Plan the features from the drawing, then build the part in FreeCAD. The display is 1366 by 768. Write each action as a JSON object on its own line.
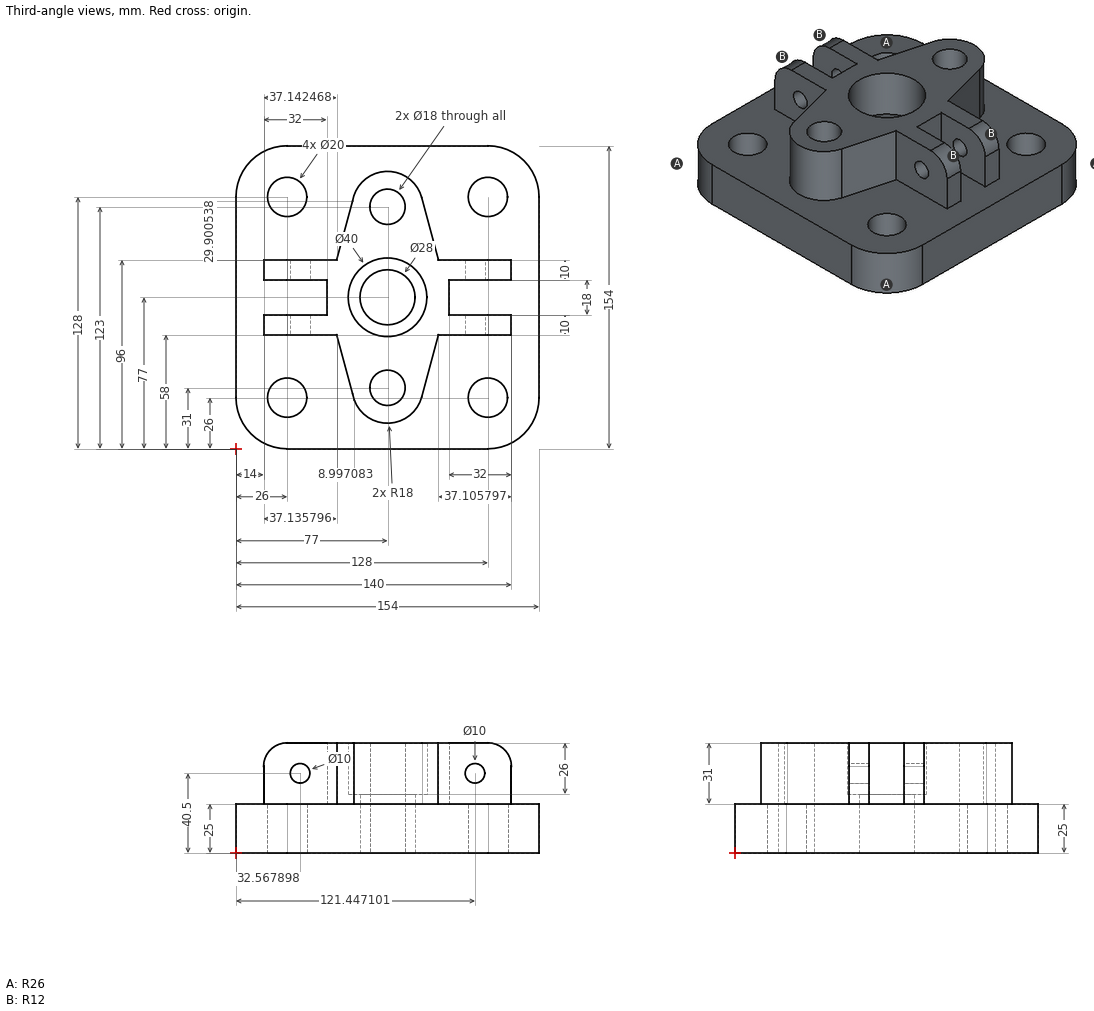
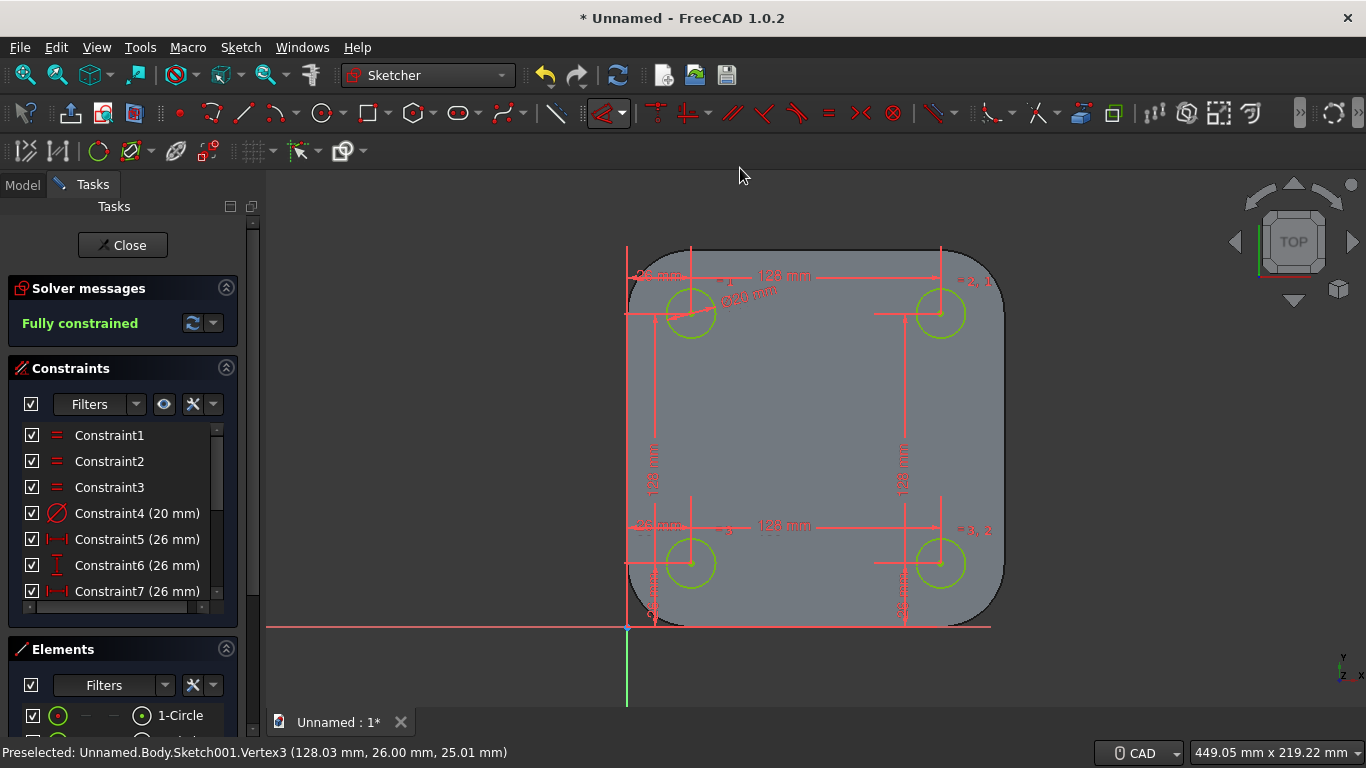
{"action": "left_click", "coordinate": [123, 245]}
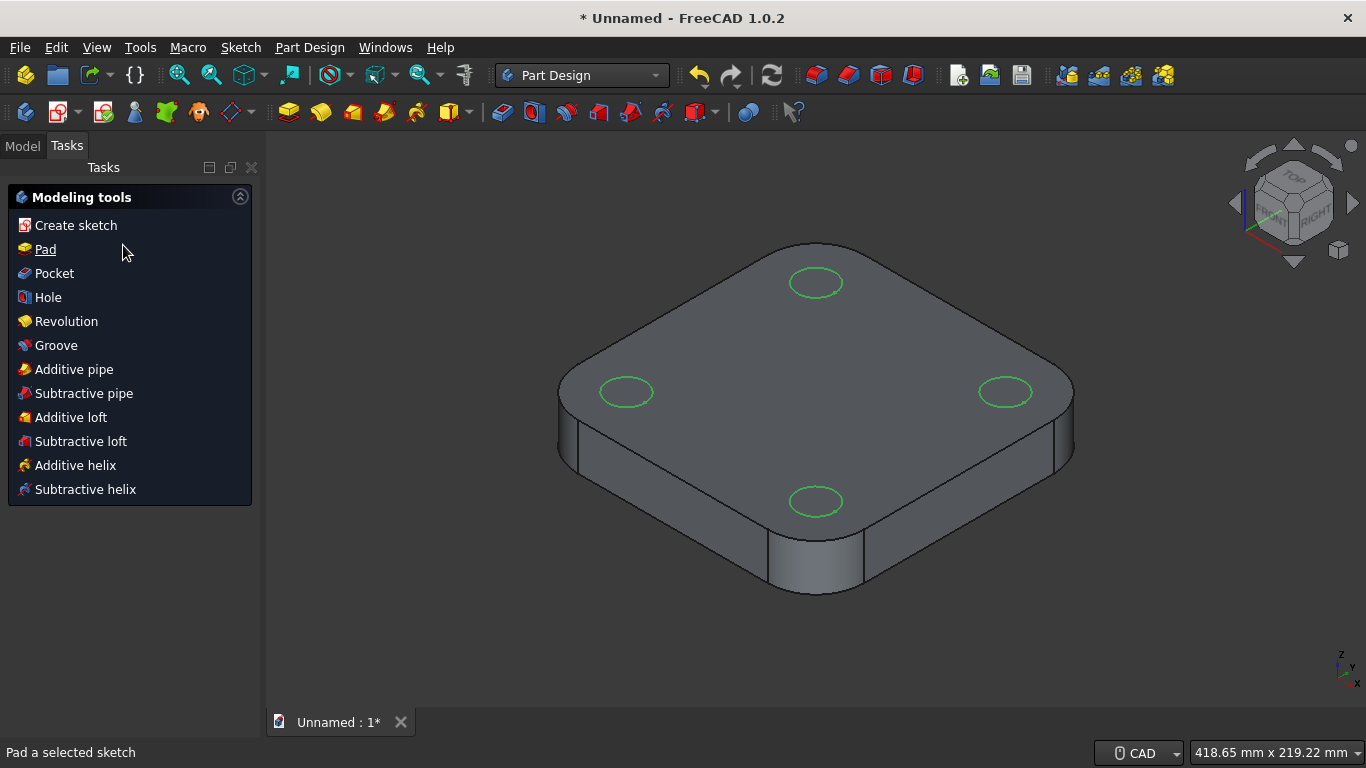
{"action": "left_click", "coordinate": [504, 112]}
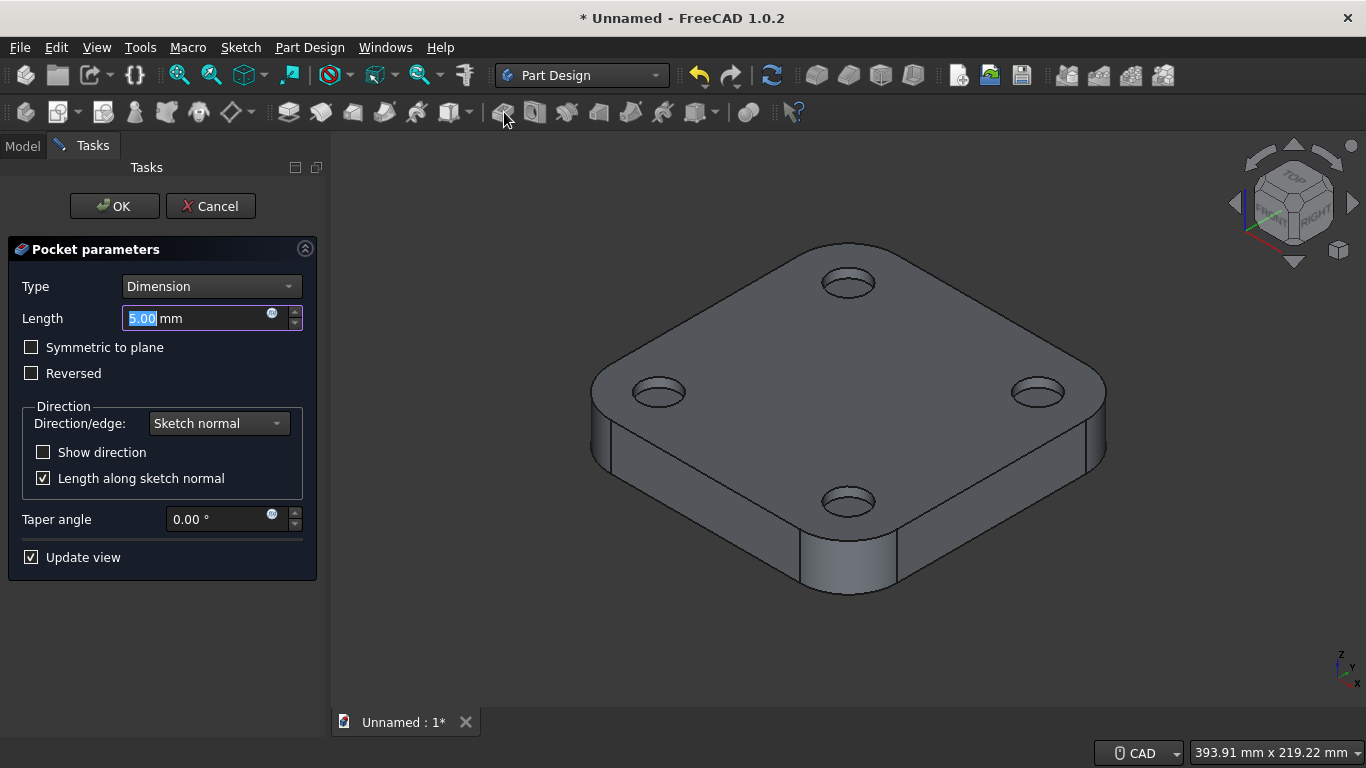
{"action": "type", "text": "25"}
{"action": "key", "text": "Tab"}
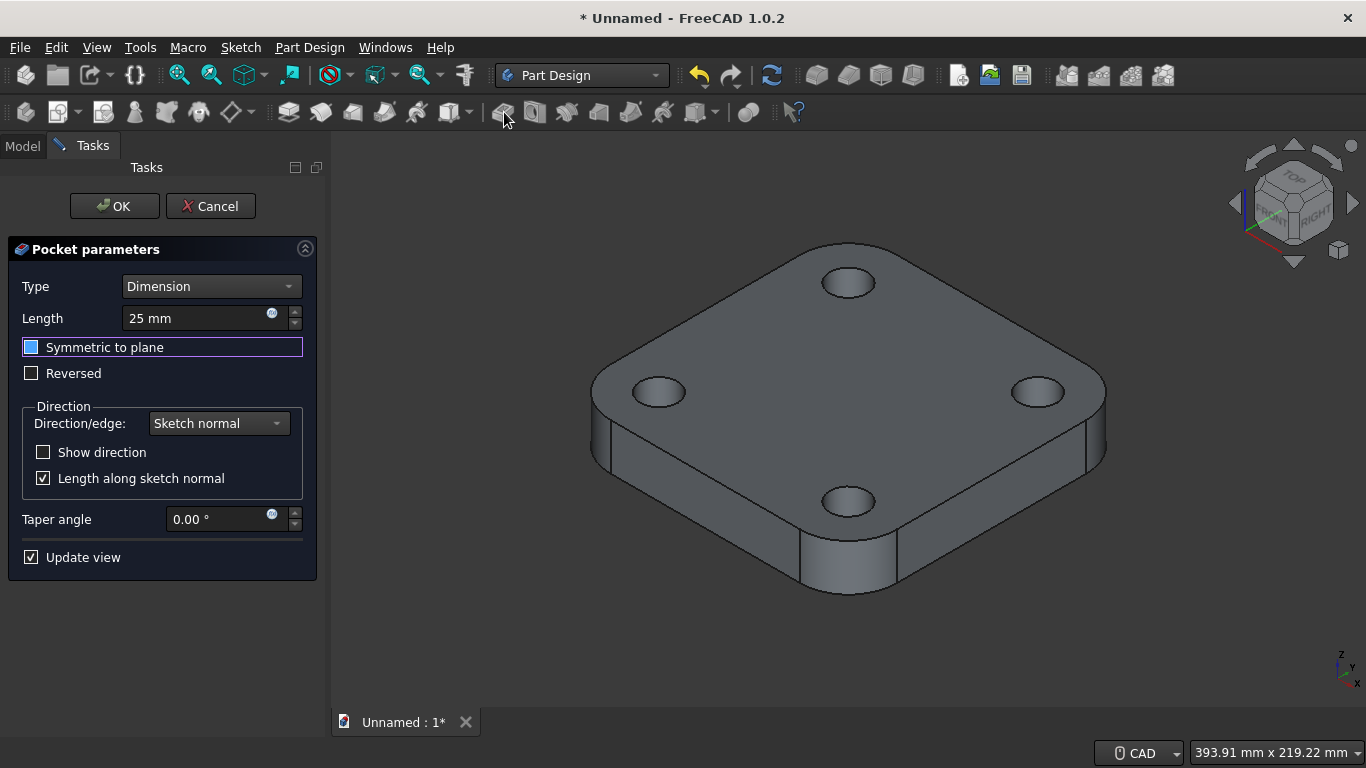
{"action": "left_click", "coordinate": [115, 206]}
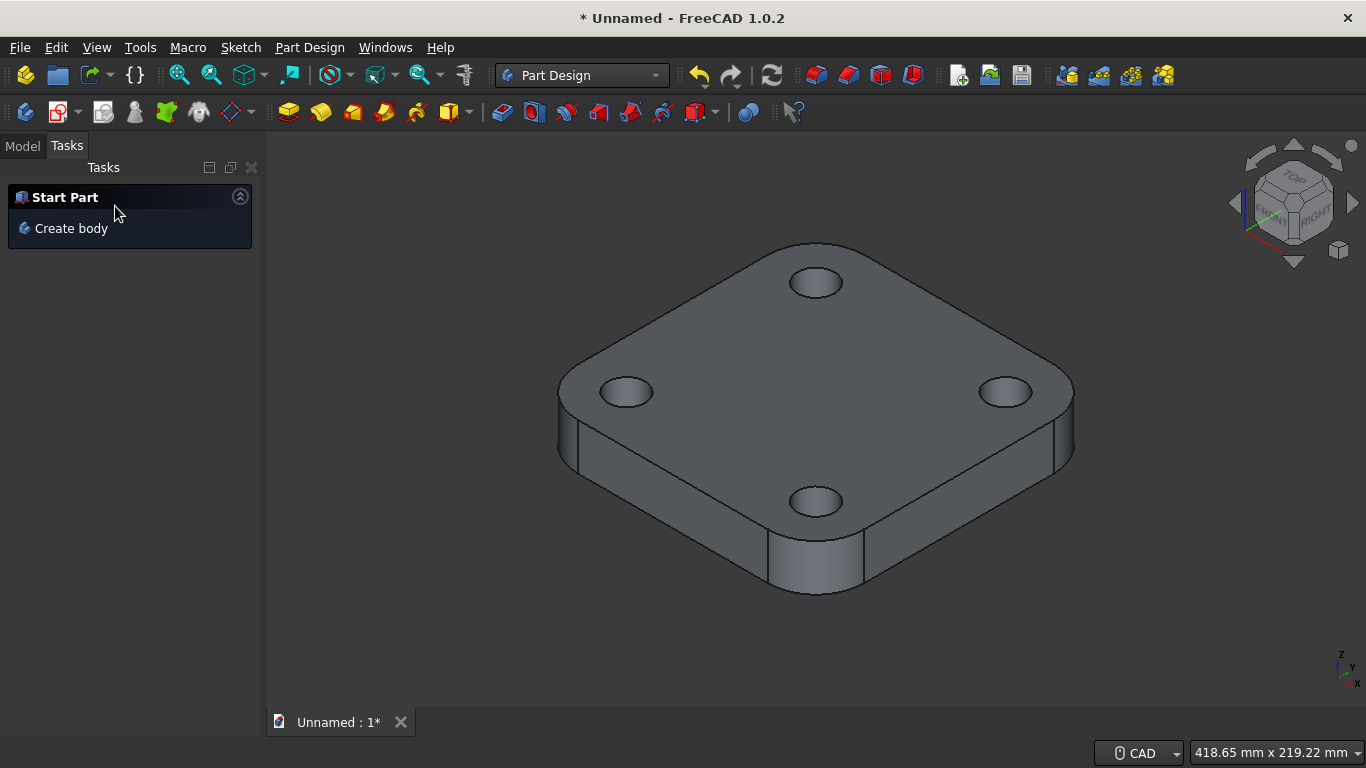
{"action": "left_click", "coordinate": [816, 391]}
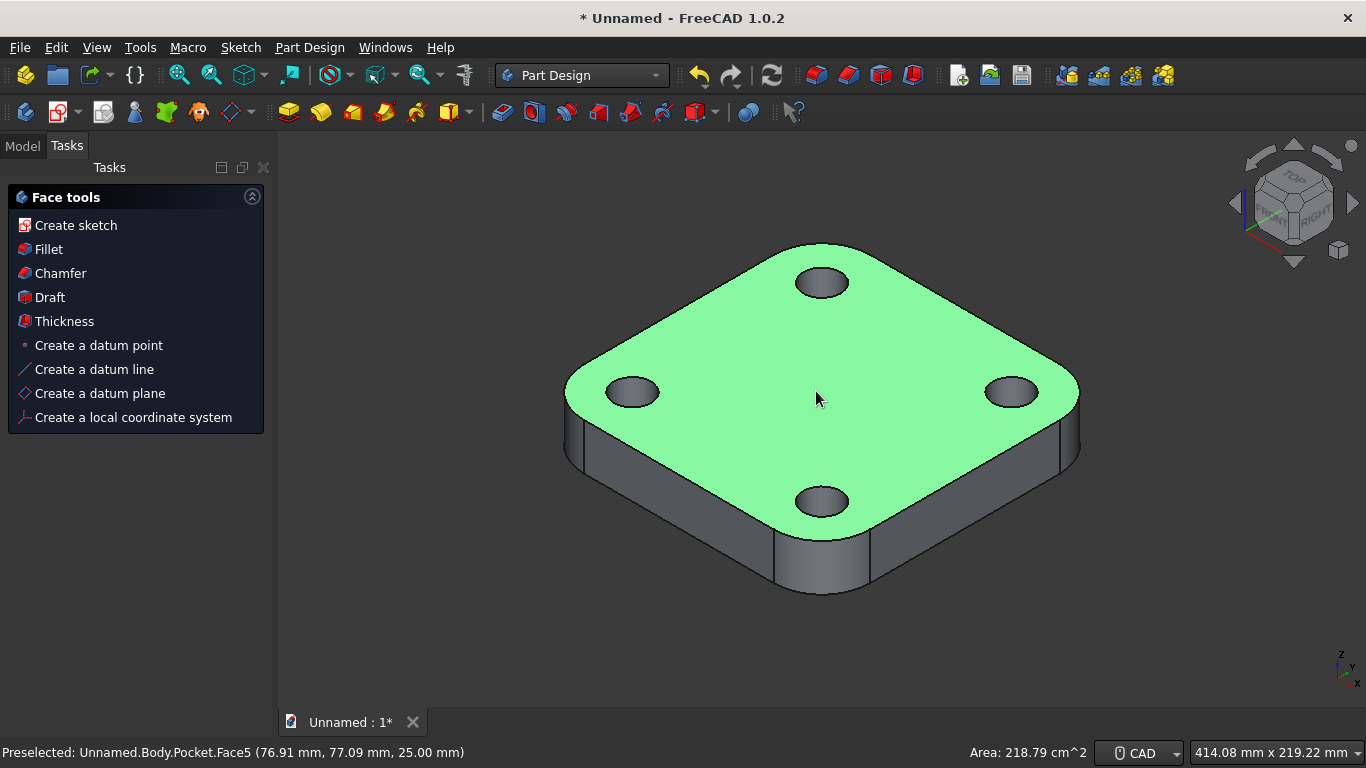
{"action": "left_click", "coordinate": [58, 112]}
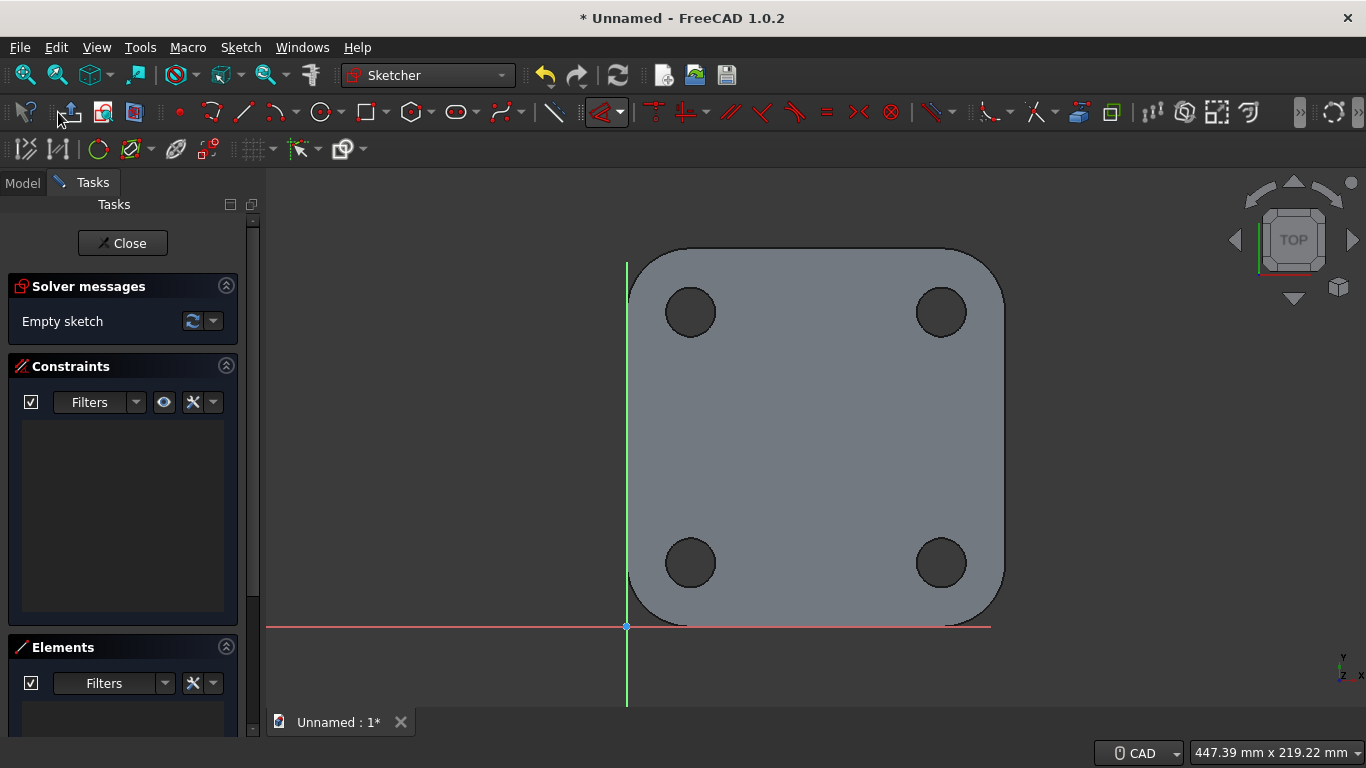
{"action": "left_click", "coordinate": [212, 112]}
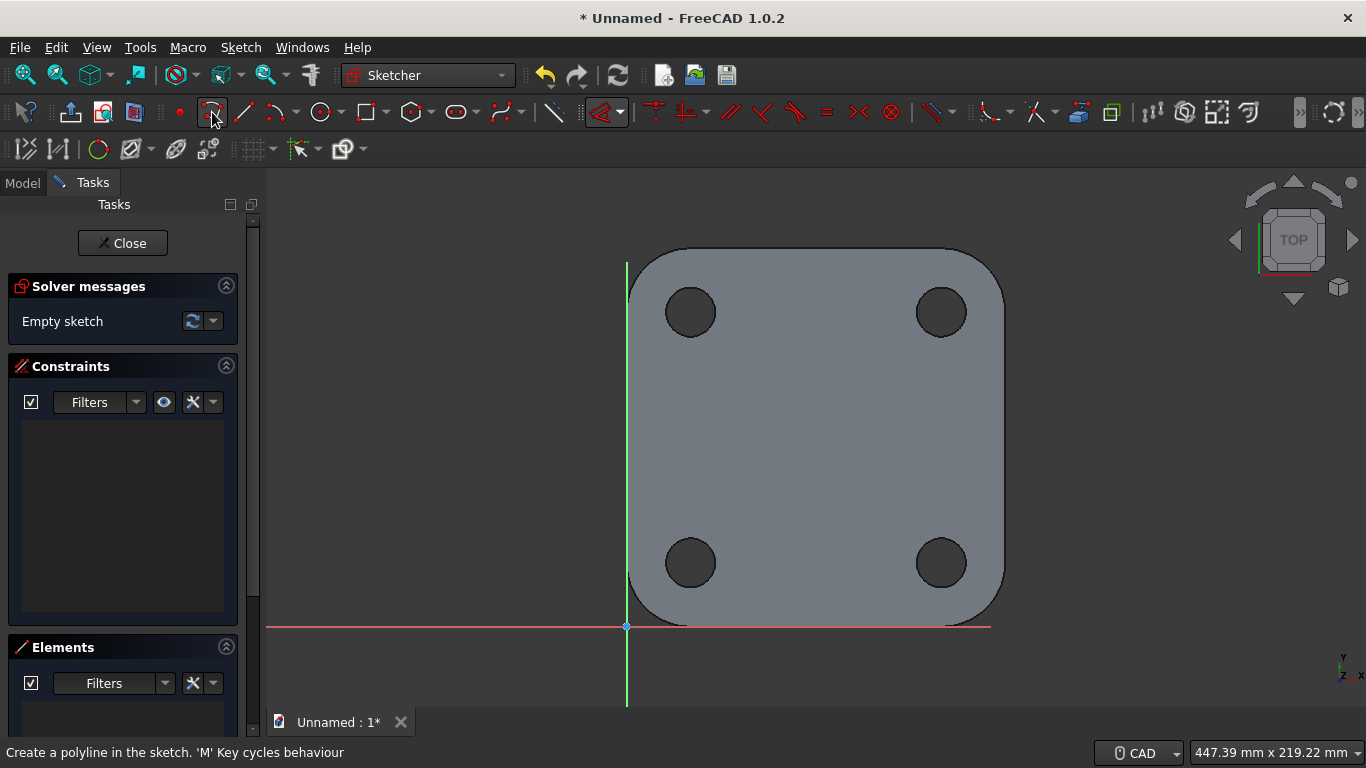
{"action": "left_click", "coordinate": [859, 562]}
{"action": "left_click", "coordinate": [880, 484]}
{"action": "left_click", "coordinate": [971, 484]}
{"action": "left_click", "coordinate": [971, 460]}
{"action": "left_click", "coordinate": [892, 460]}
{"action": "left_click", "coordinate": [892, 415]}
{"action": "left_click", "coordinate": [971, 415]}
{"action": "left_click", "coordinate": [971, 391]}
{"action": "left_click", "coordinate": [880, 391]}
{"action": "left_click", "coordinate": [859, 313]}
{"action": "right_click", "coordinate": [859, 313]}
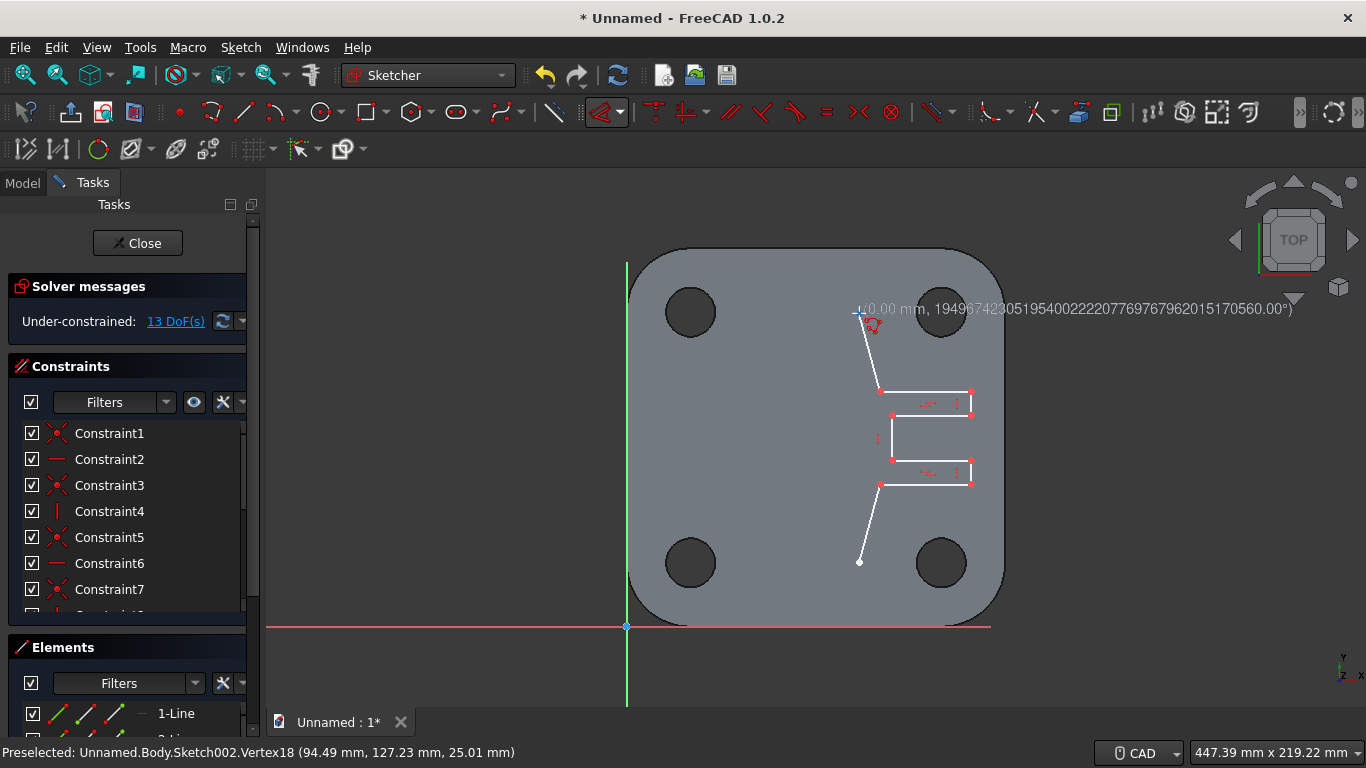
{"action": "left_click", "coordinate": [772, 317]}
{"action": "left_click", "coordinate": [752, 391]}
{"action": "left_click", "coordinate": [661, 391]}
{"action": "left_click", "coordinate": [661, 415]}
{"action": "left_click", "coordinate": [740, 415]}
{"action": "left_click", "coordinate": [740, 460]}
{"action": "left_click", "coordinate": [661, 460]}
{"action": "left_click", "coordinate": [661, 484]}
{"action": "left_click", "coordinate": [752, 484]}
{"action": "left_click", "coordinate": [775, 566]}
{"action": "right_click", "coordinate": [775, 566]}